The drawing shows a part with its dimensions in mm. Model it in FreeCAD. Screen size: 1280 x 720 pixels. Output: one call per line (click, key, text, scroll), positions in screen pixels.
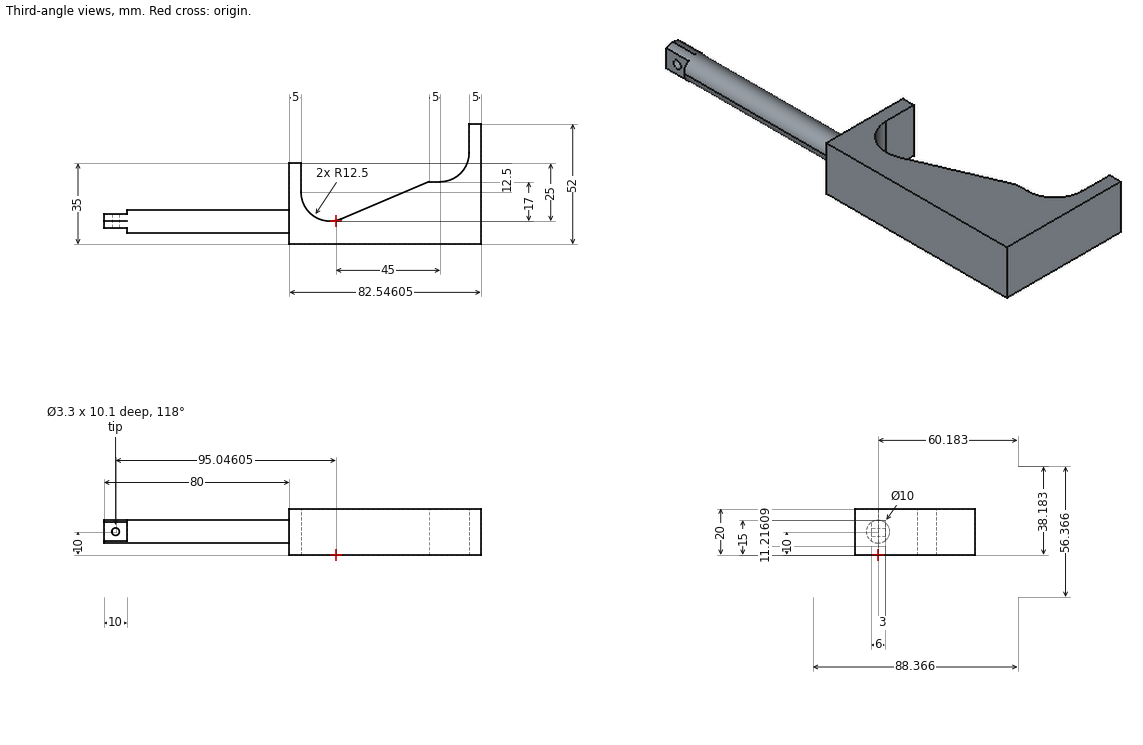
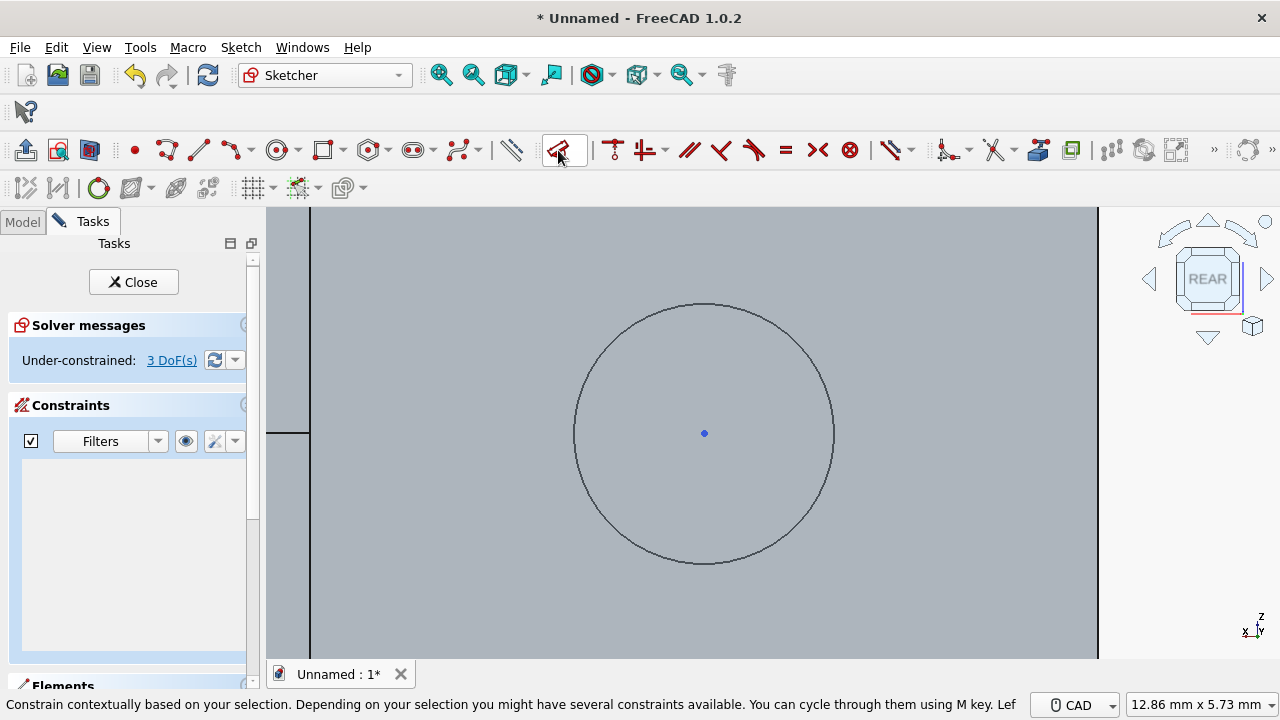
click(796, 342)
click(819, 319)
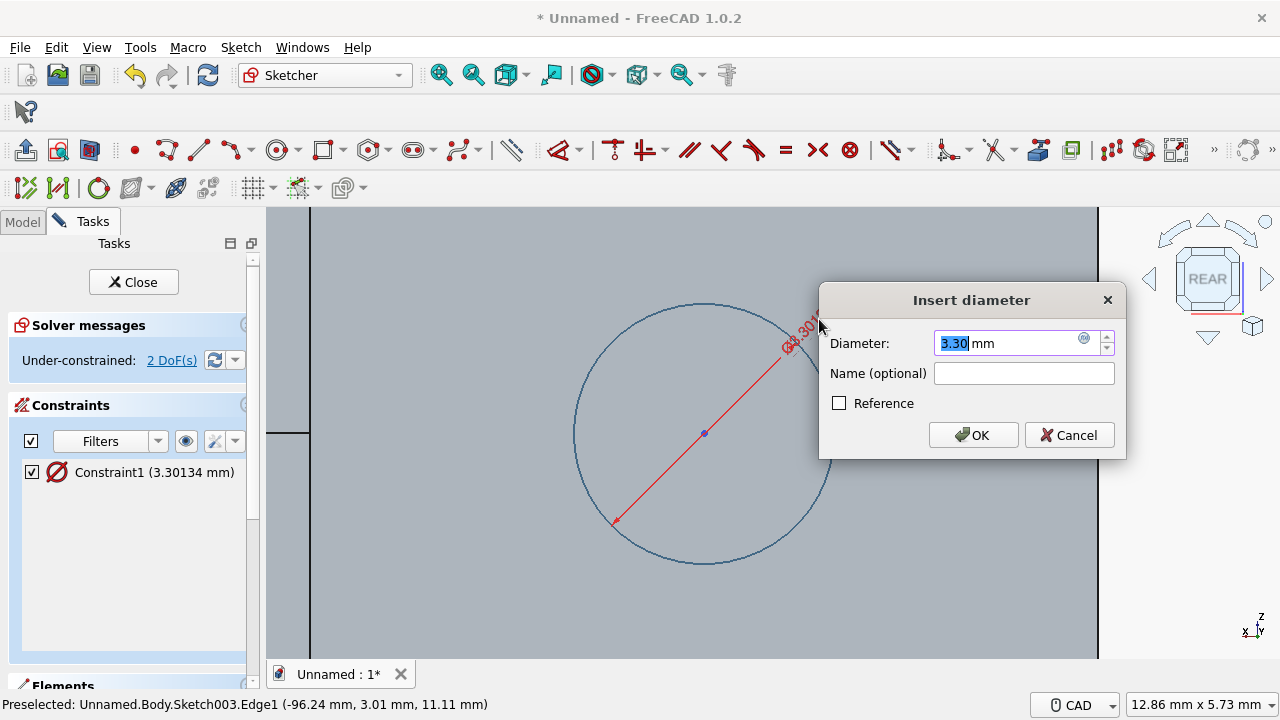
text(3.3)
key(Return)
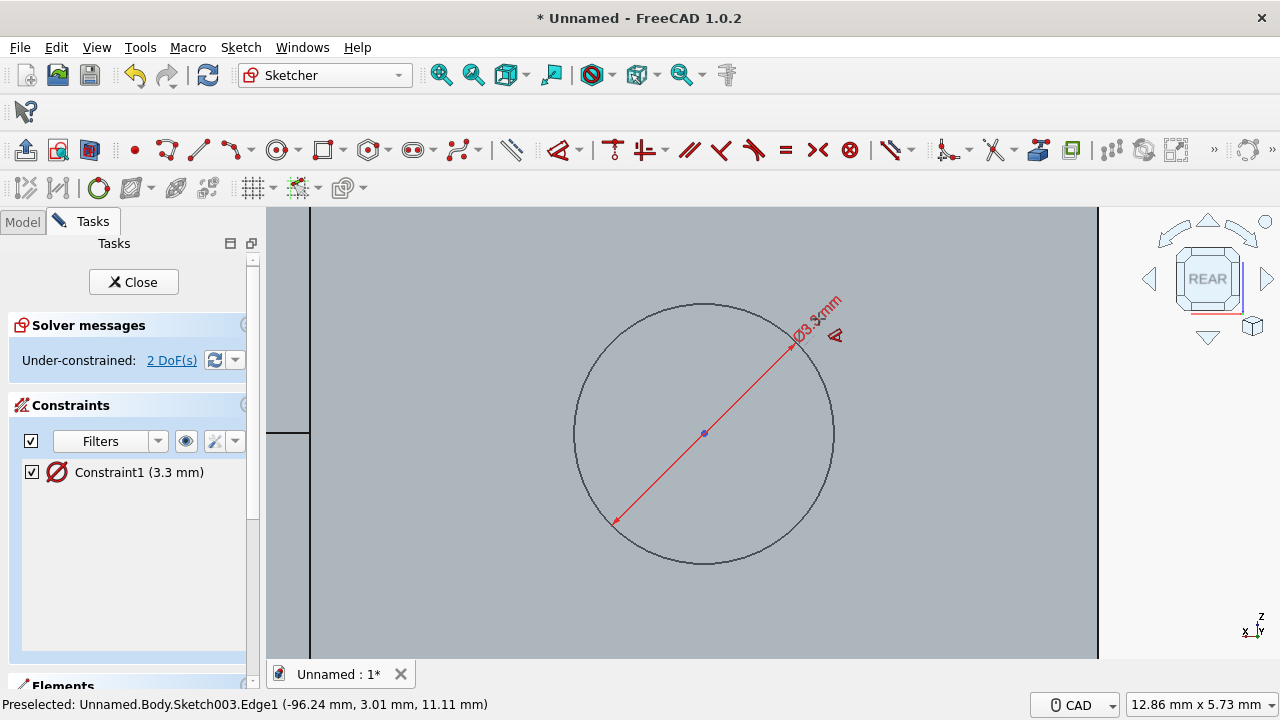
click(704, 434)
click(738, 532)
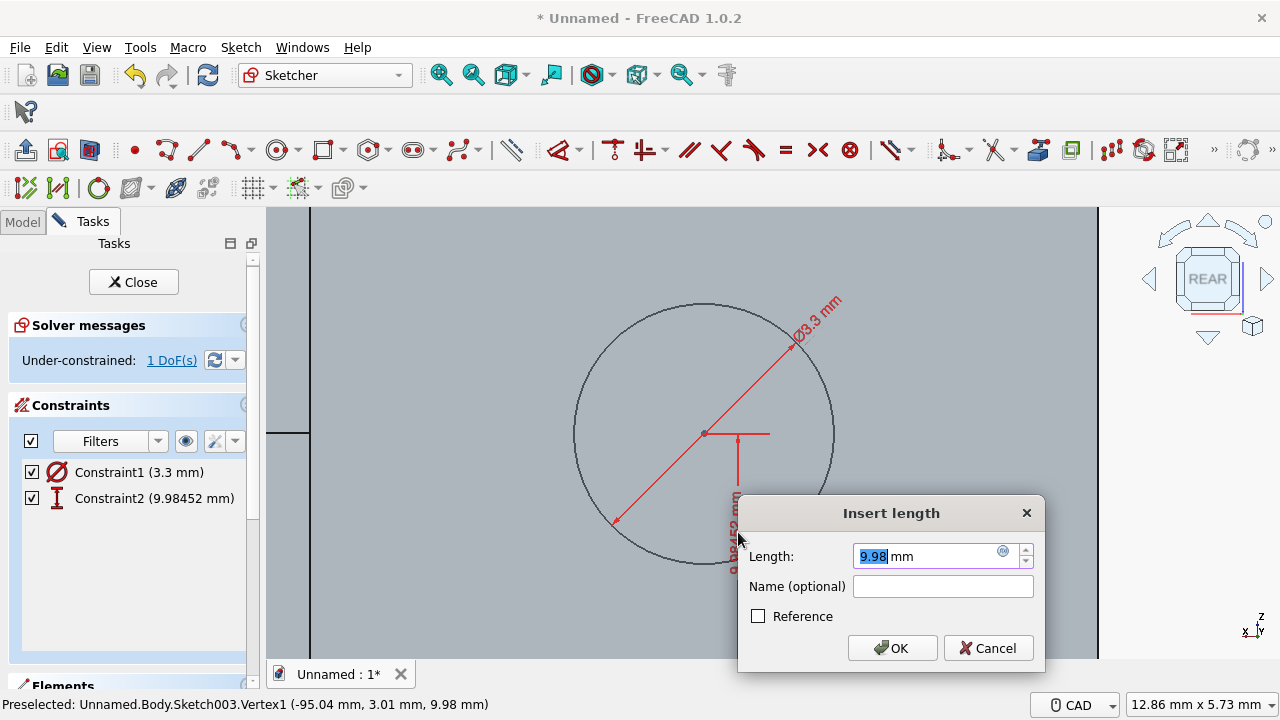
text(10)
key(Return)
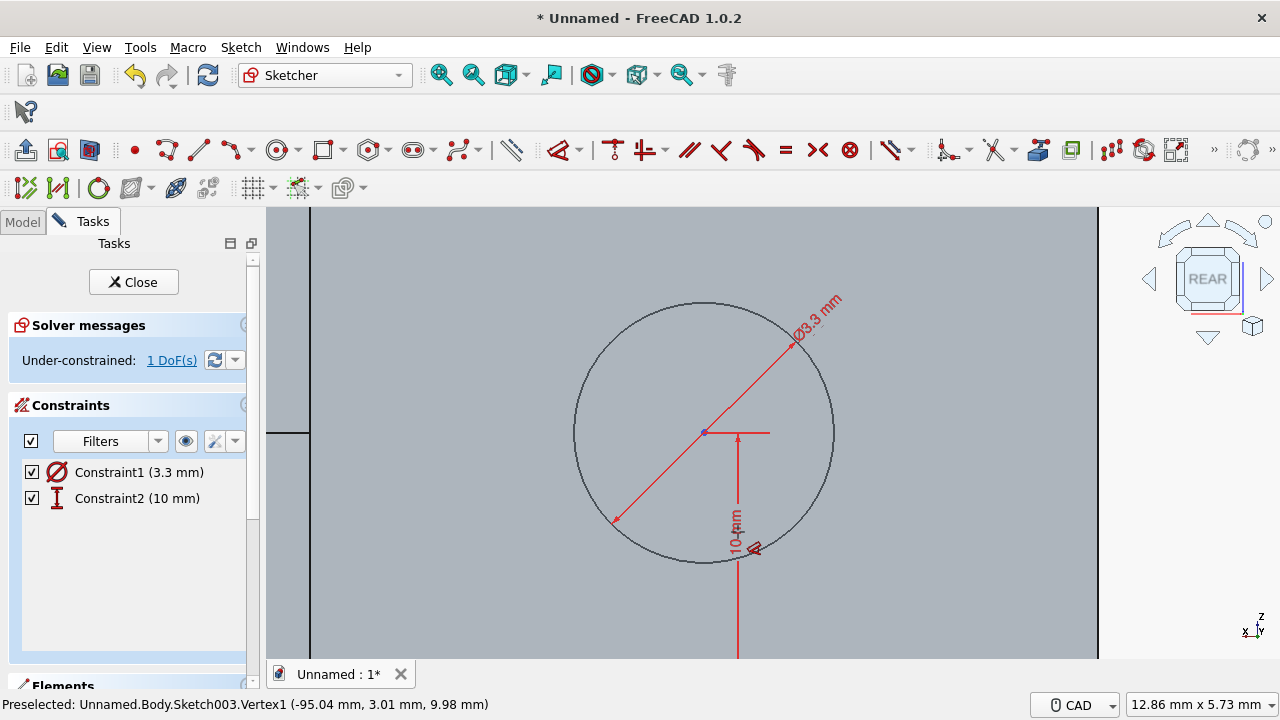
click(704, 433)
click(499, 399)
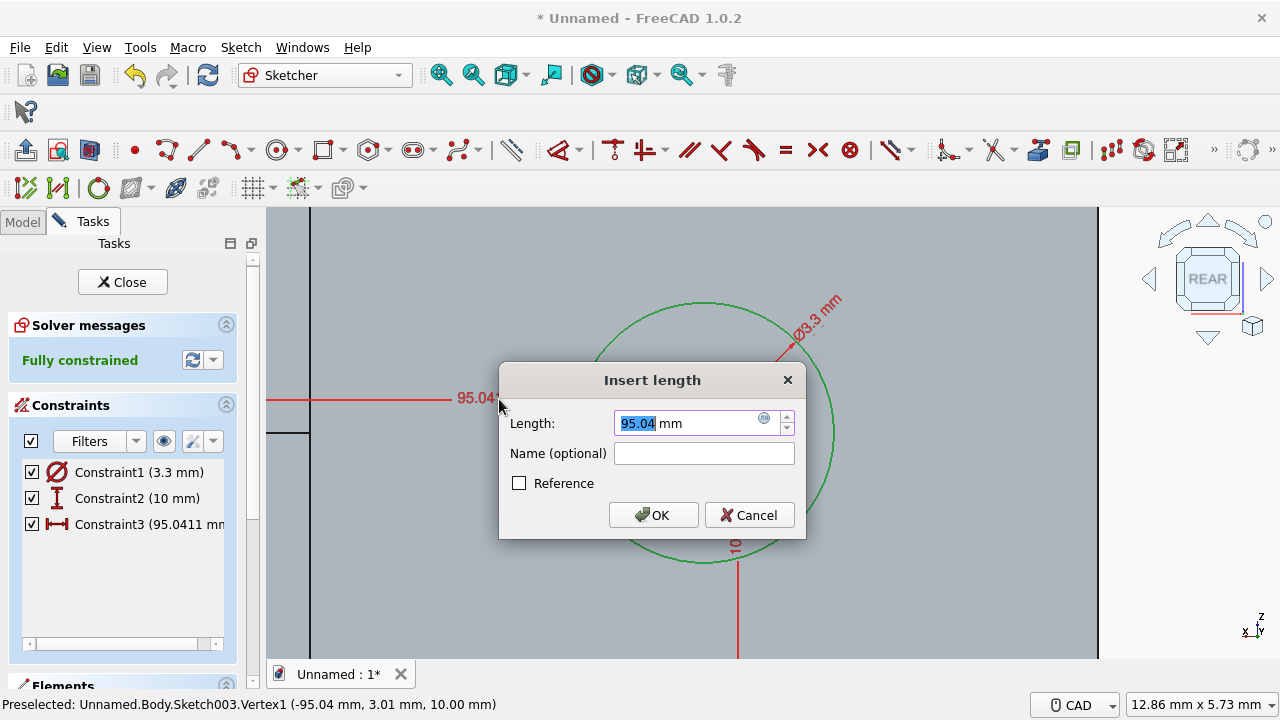
text(95.04605)
key(Return)
key(Escape)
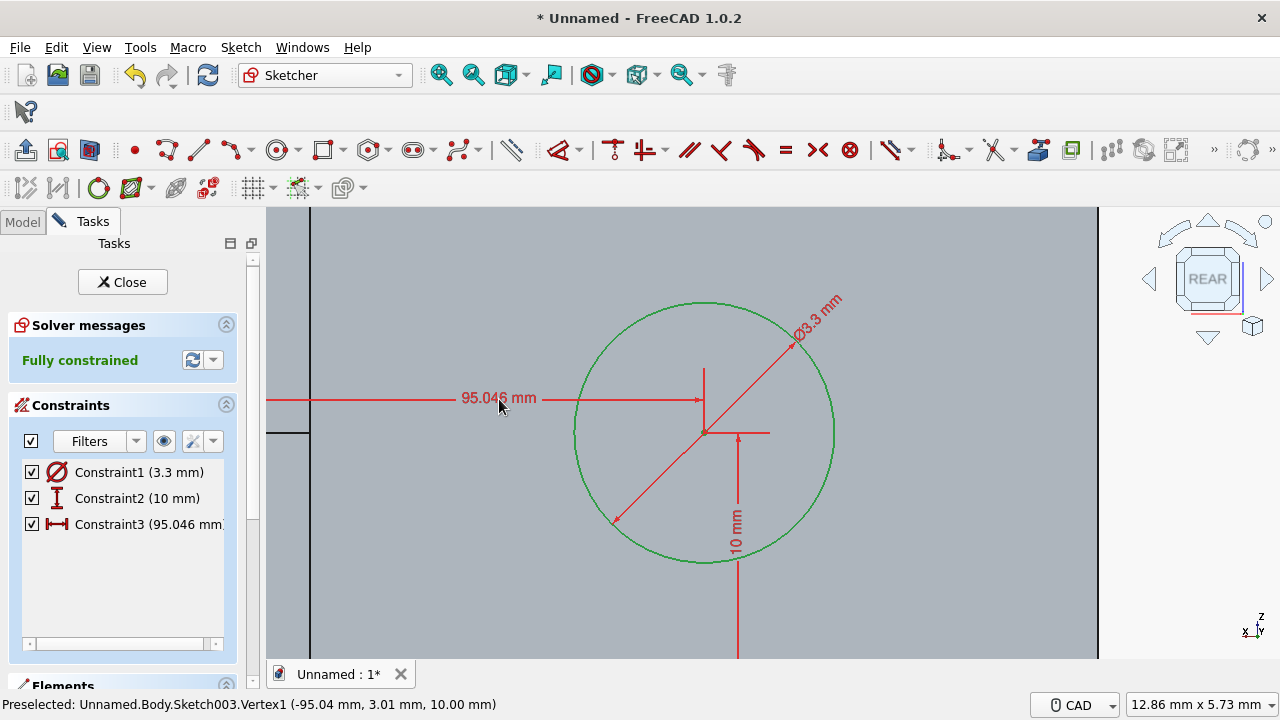
click(123, 282)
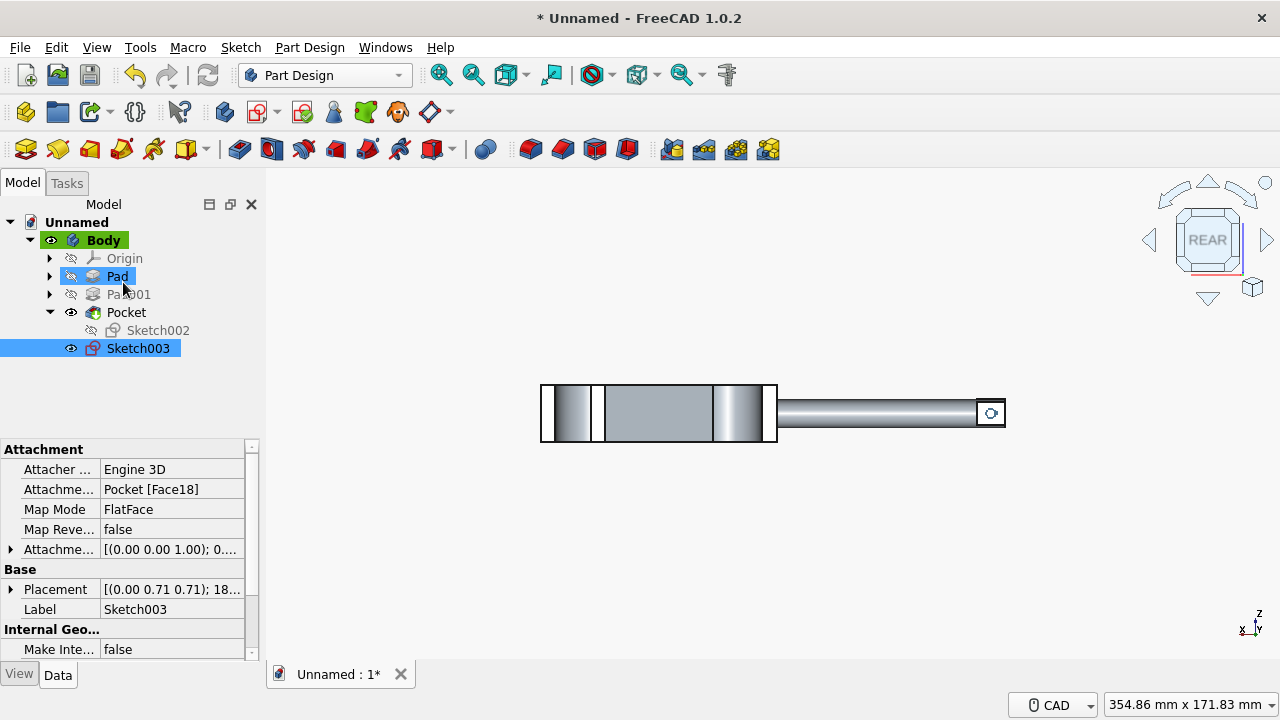
click(272, 150)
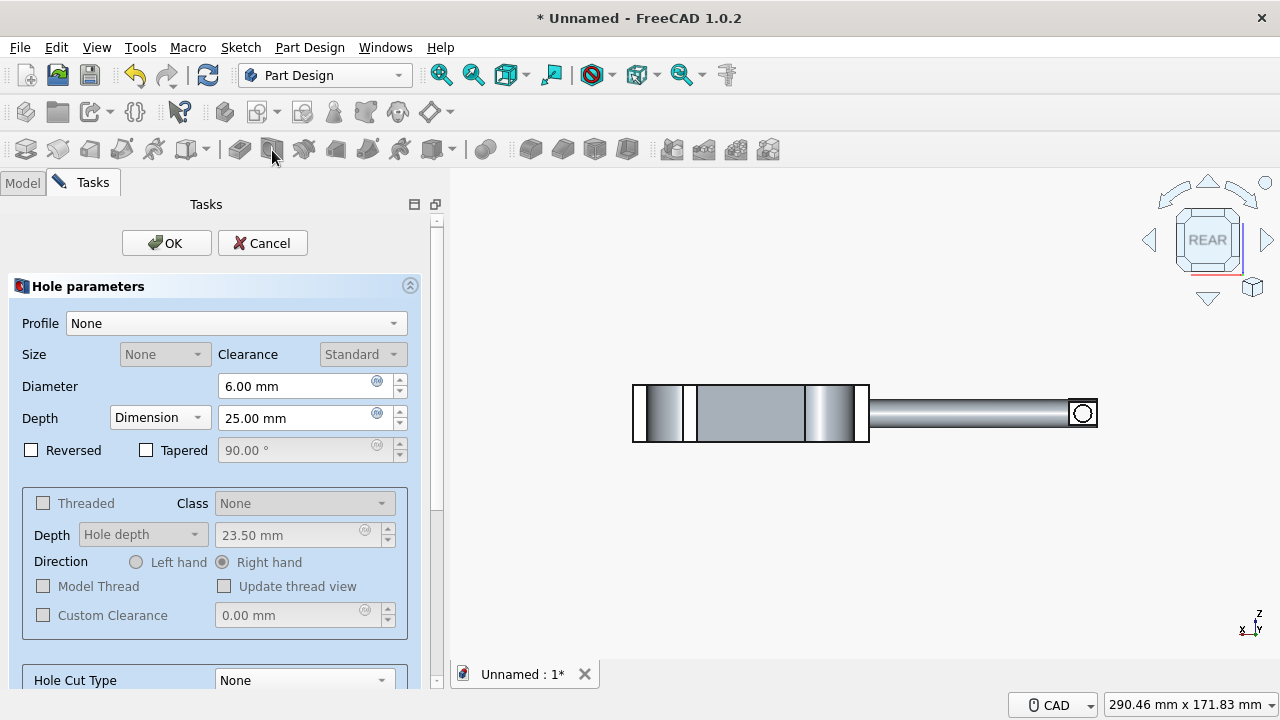
triple_click(305, 386)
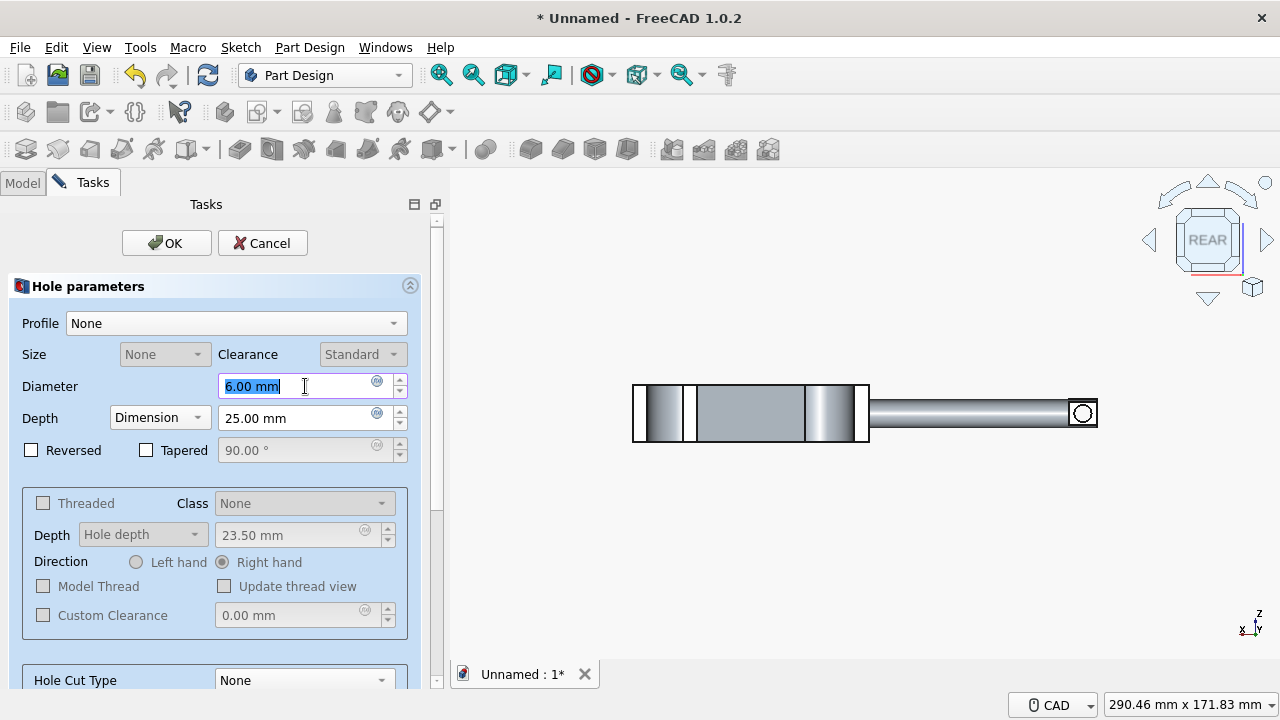
text(3.3)
key(Tab)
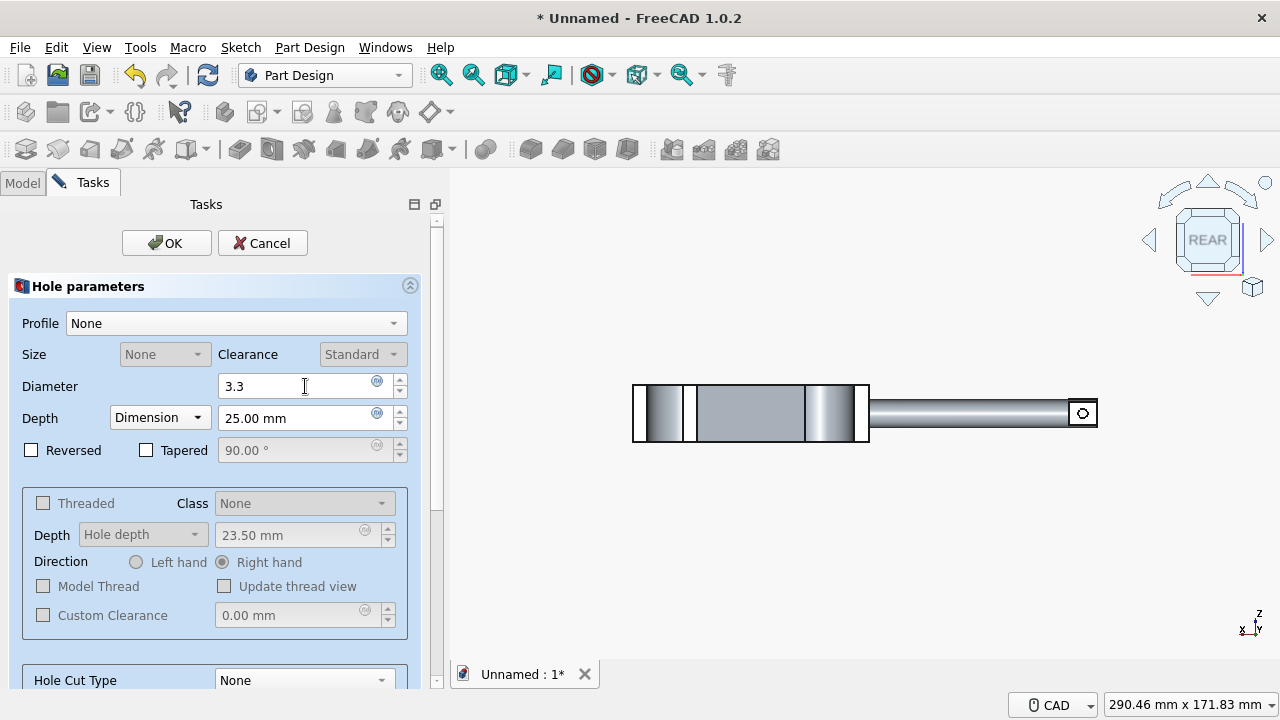
triple_click(305, 418)